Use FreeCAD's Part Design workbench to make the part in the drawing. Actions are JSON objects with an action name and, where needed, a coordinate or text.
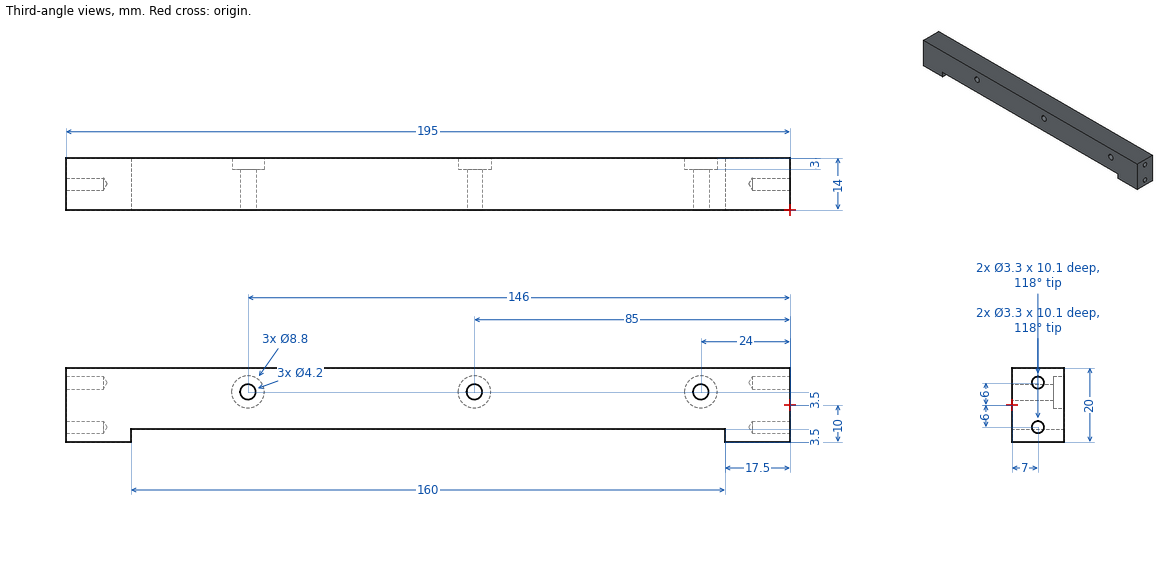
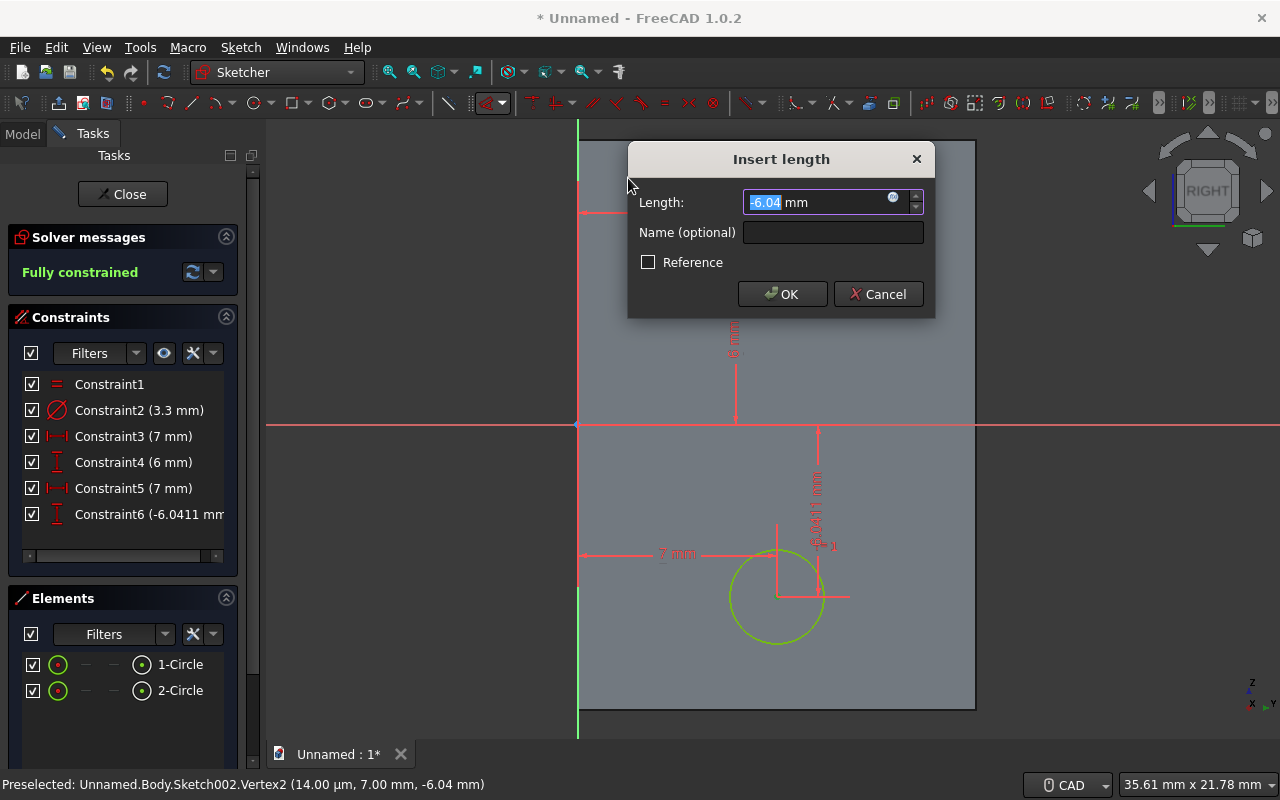
{"action": "type", "text": "-6"}
{"action": "key", "text": "Return"}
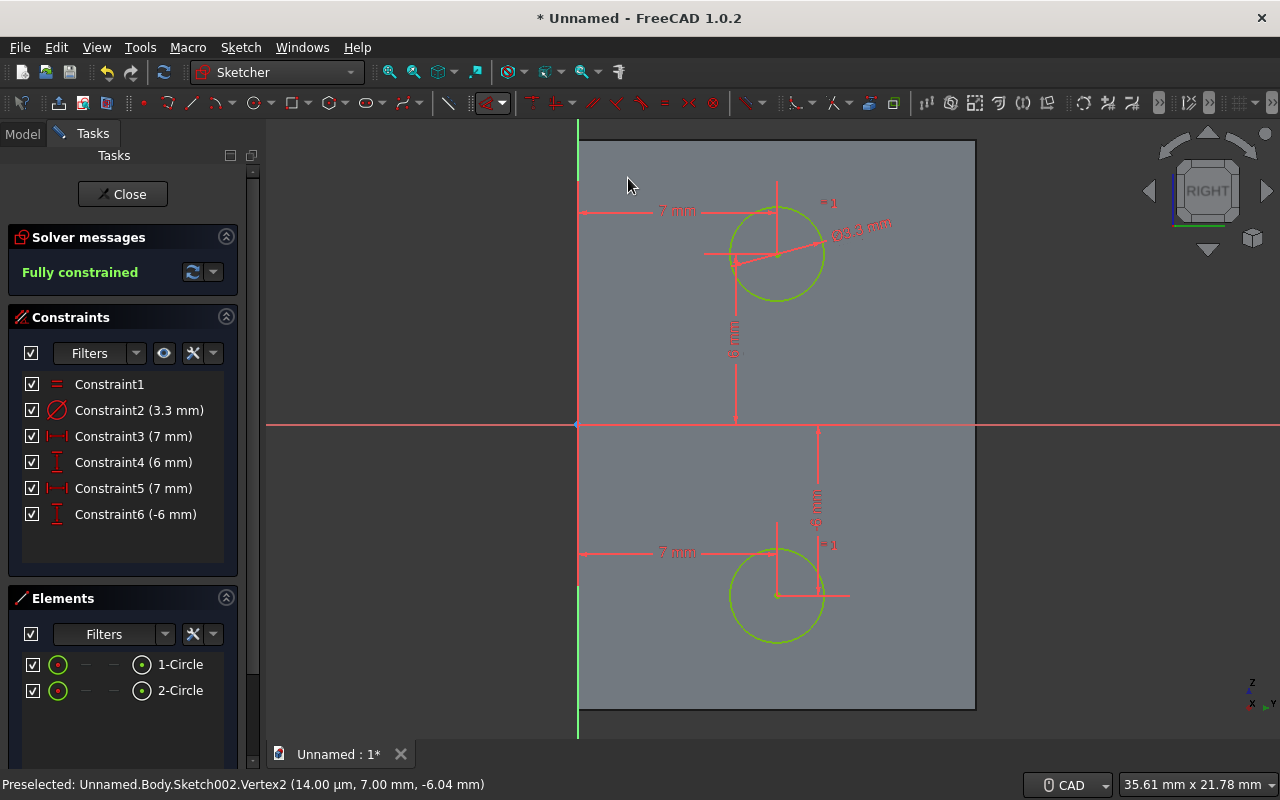
{"action": "left_click", "coordinate": [123, 194]}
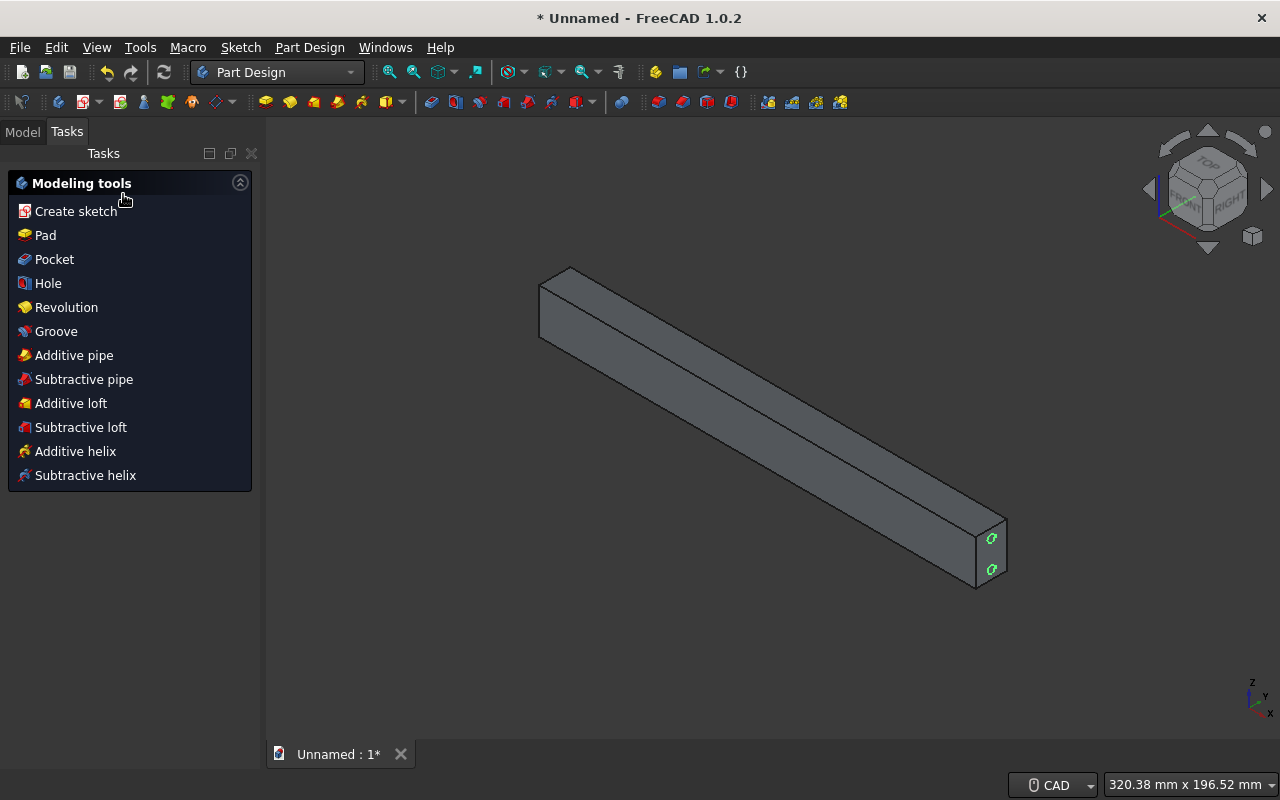
{"action": "left_click", "coordinate": [456, 102]}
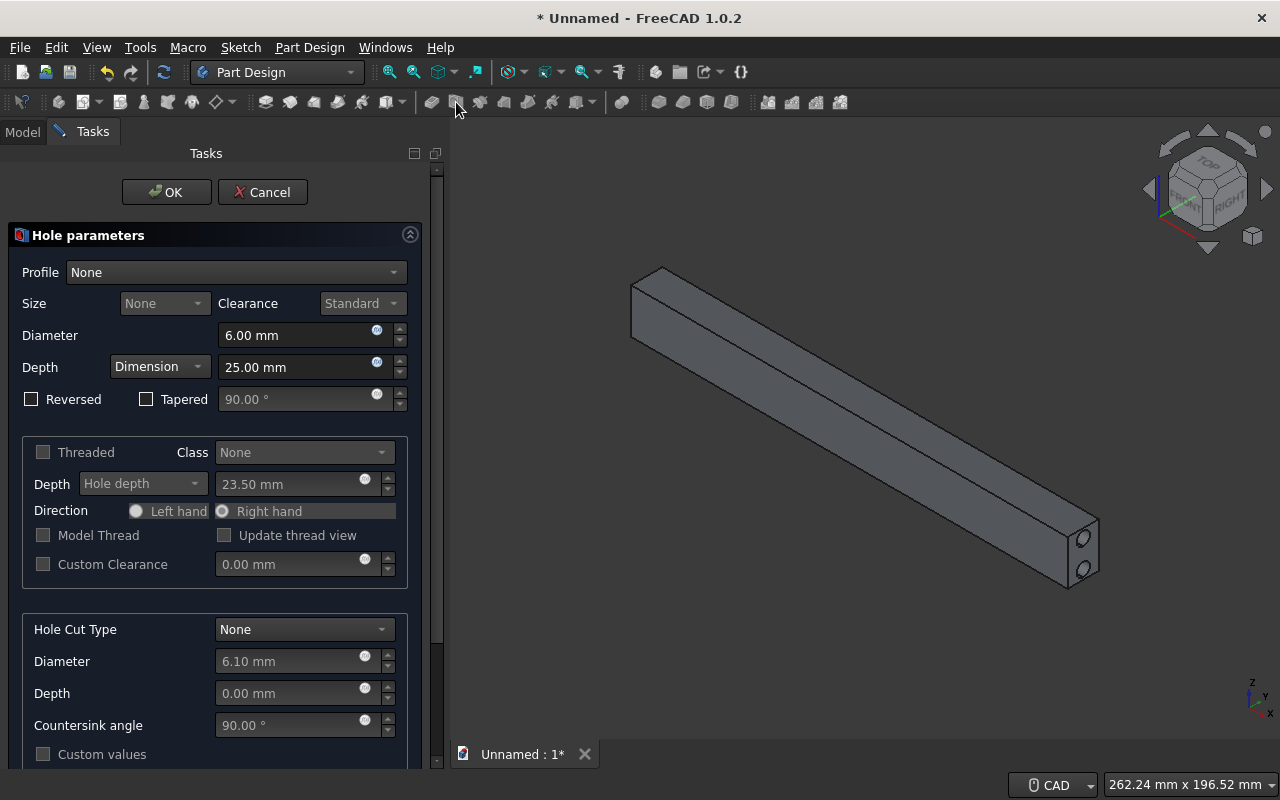
{"action": "triple_click", "coordinate": [305, 335]}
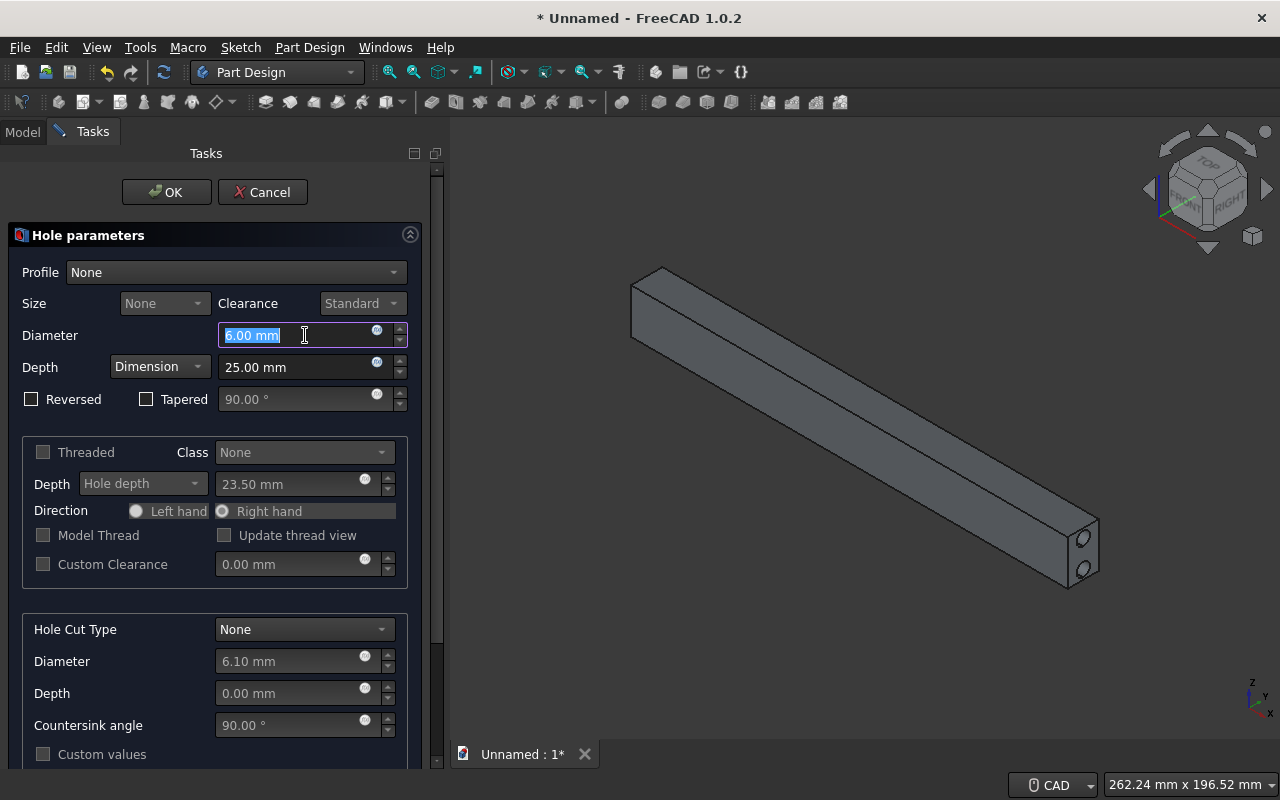
{"action": "type", "text": "3.3"}
{"action": "key", "text": "Tab"}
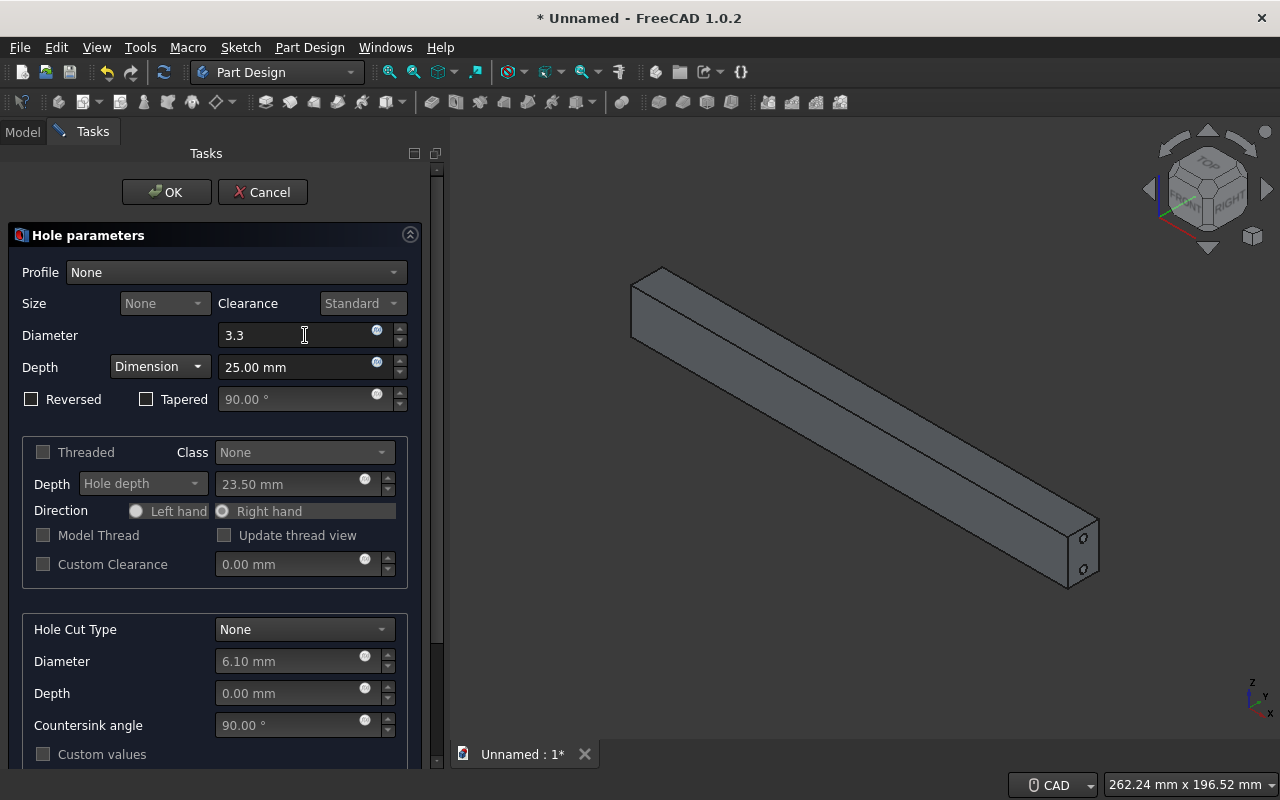
{"action": "triple_click", "coordinate": [305, 367]}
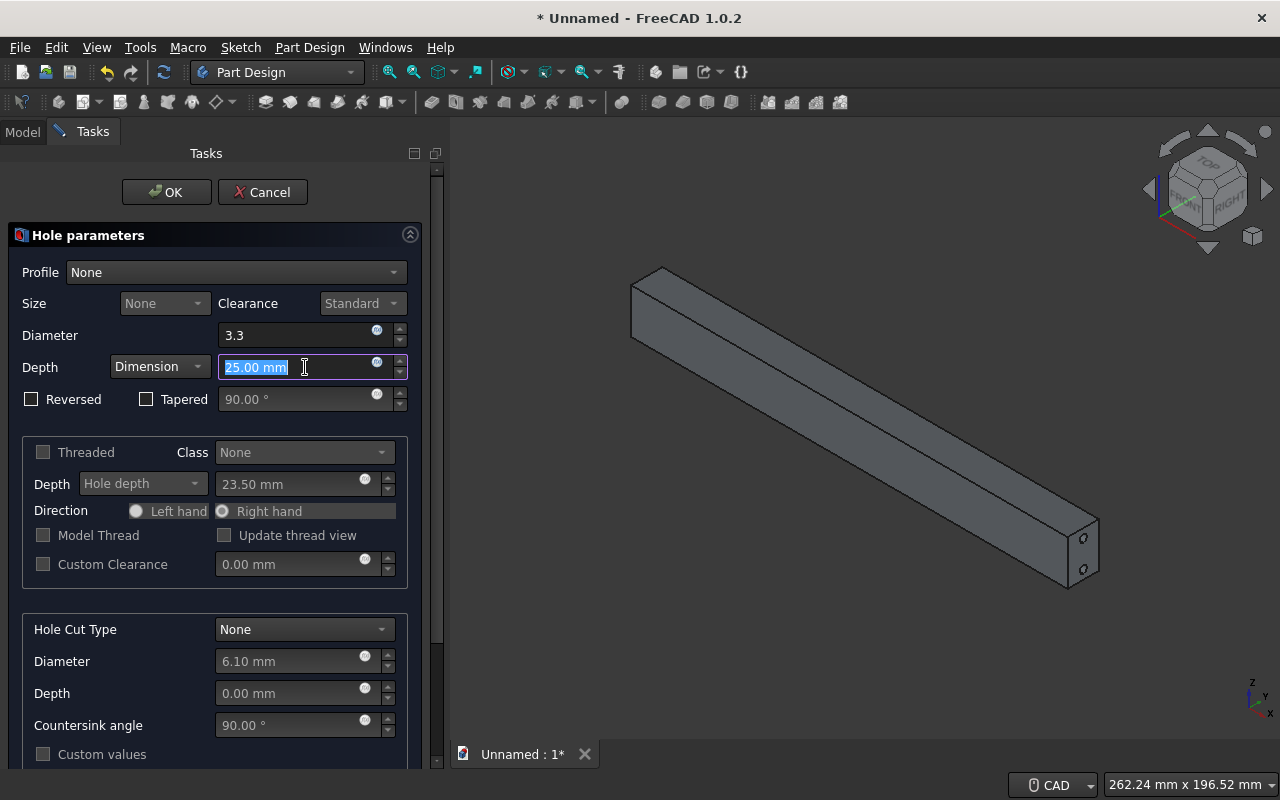
{"action": "type", "text": "10.1"}
{"action": "key", "text": "Tab"}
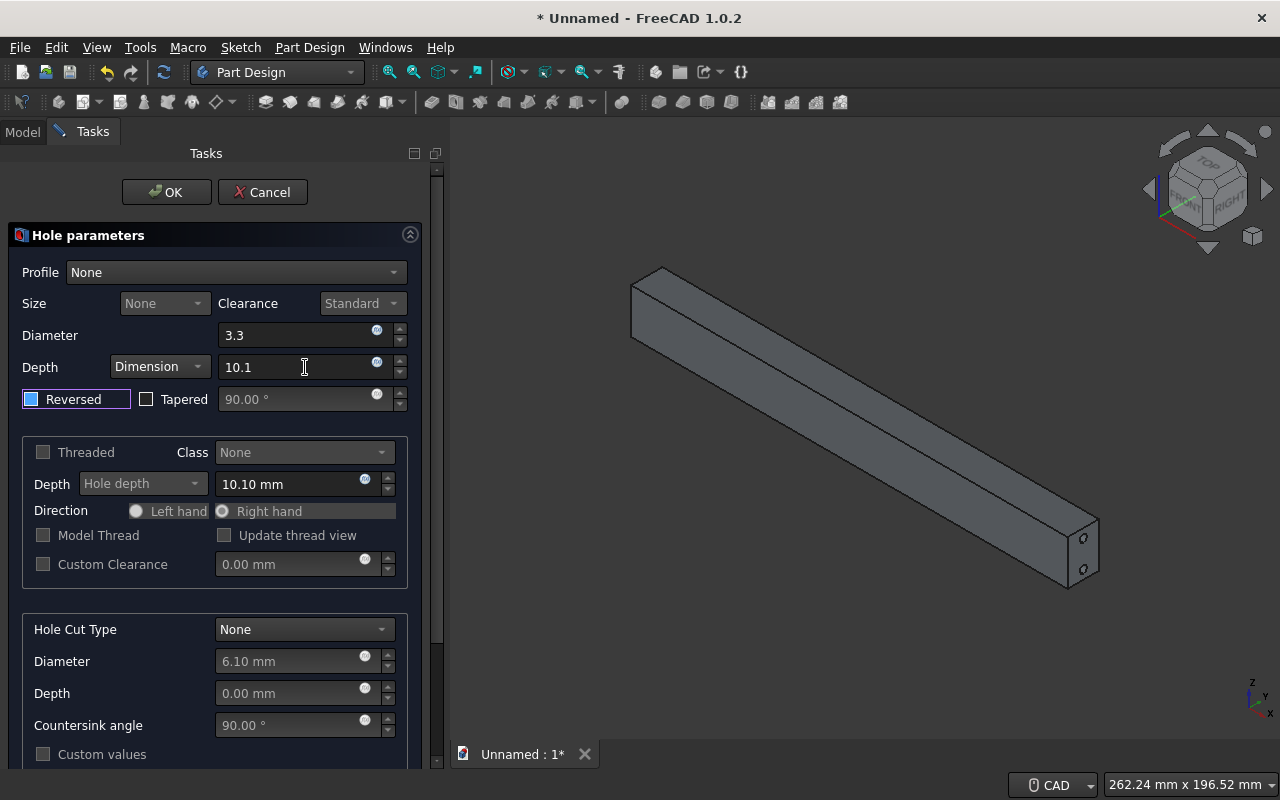
{"action": "left_click", "coordinate": [167, 192]}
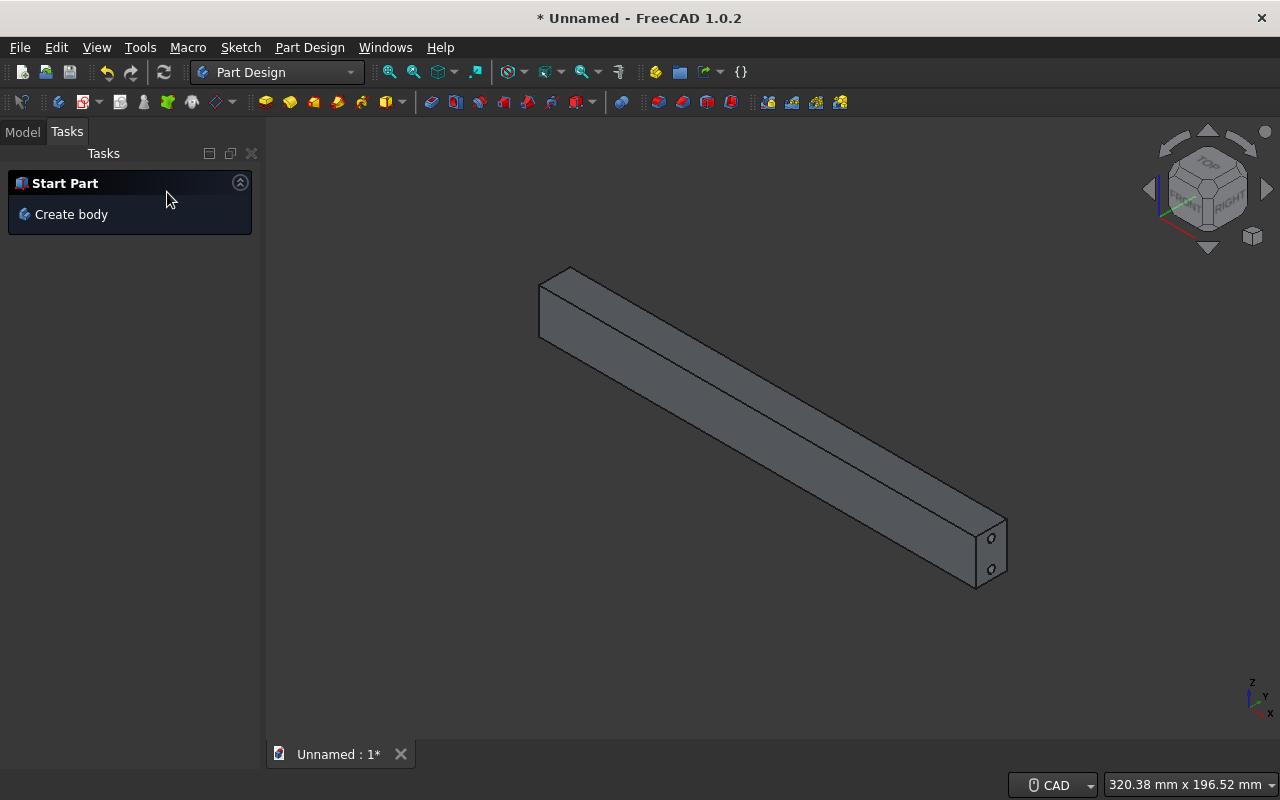
{"action": "key", "text": "4"}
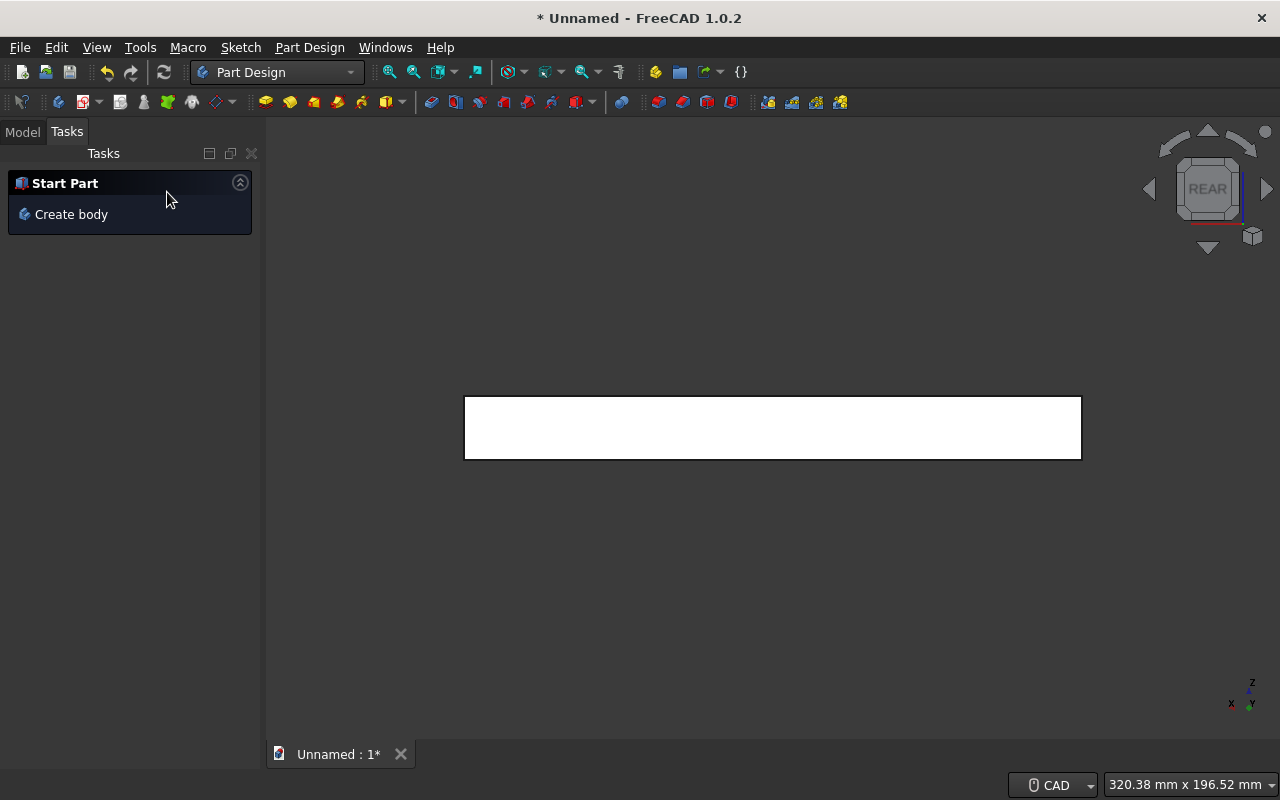
{"action": "left_click", "coordinate": [508, 427]}